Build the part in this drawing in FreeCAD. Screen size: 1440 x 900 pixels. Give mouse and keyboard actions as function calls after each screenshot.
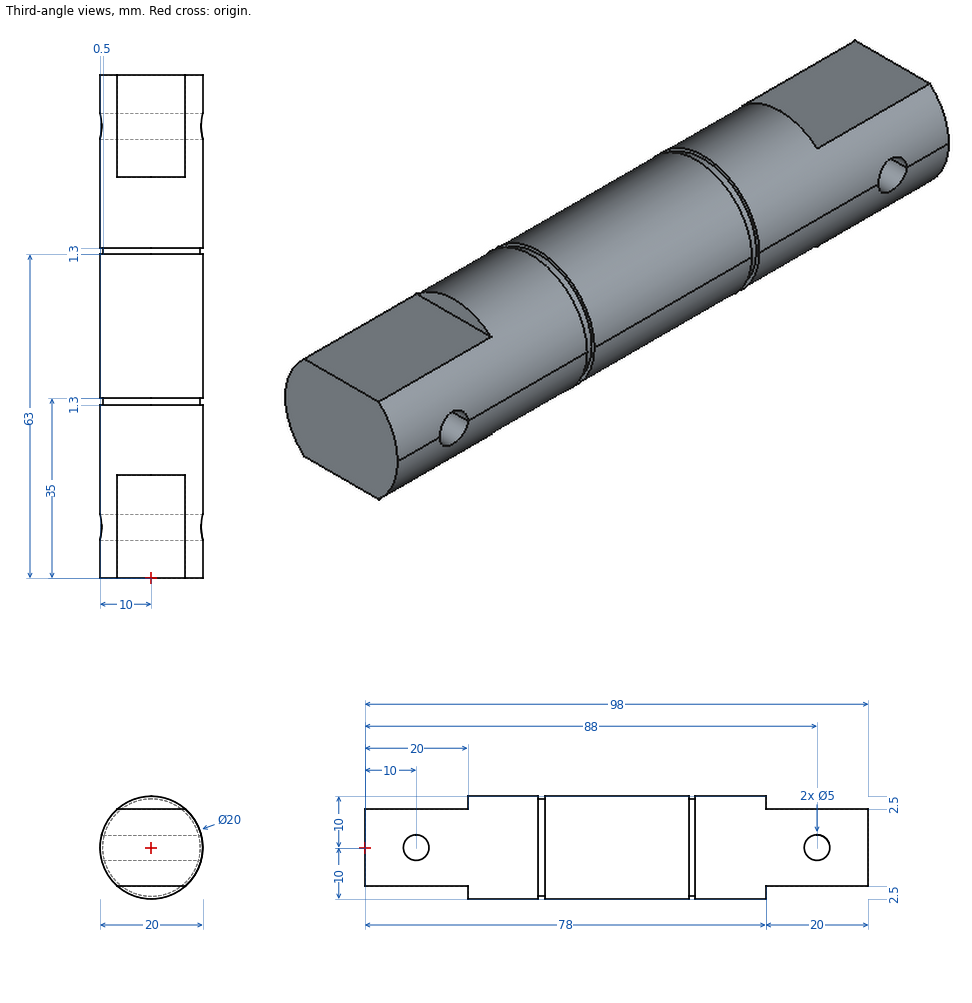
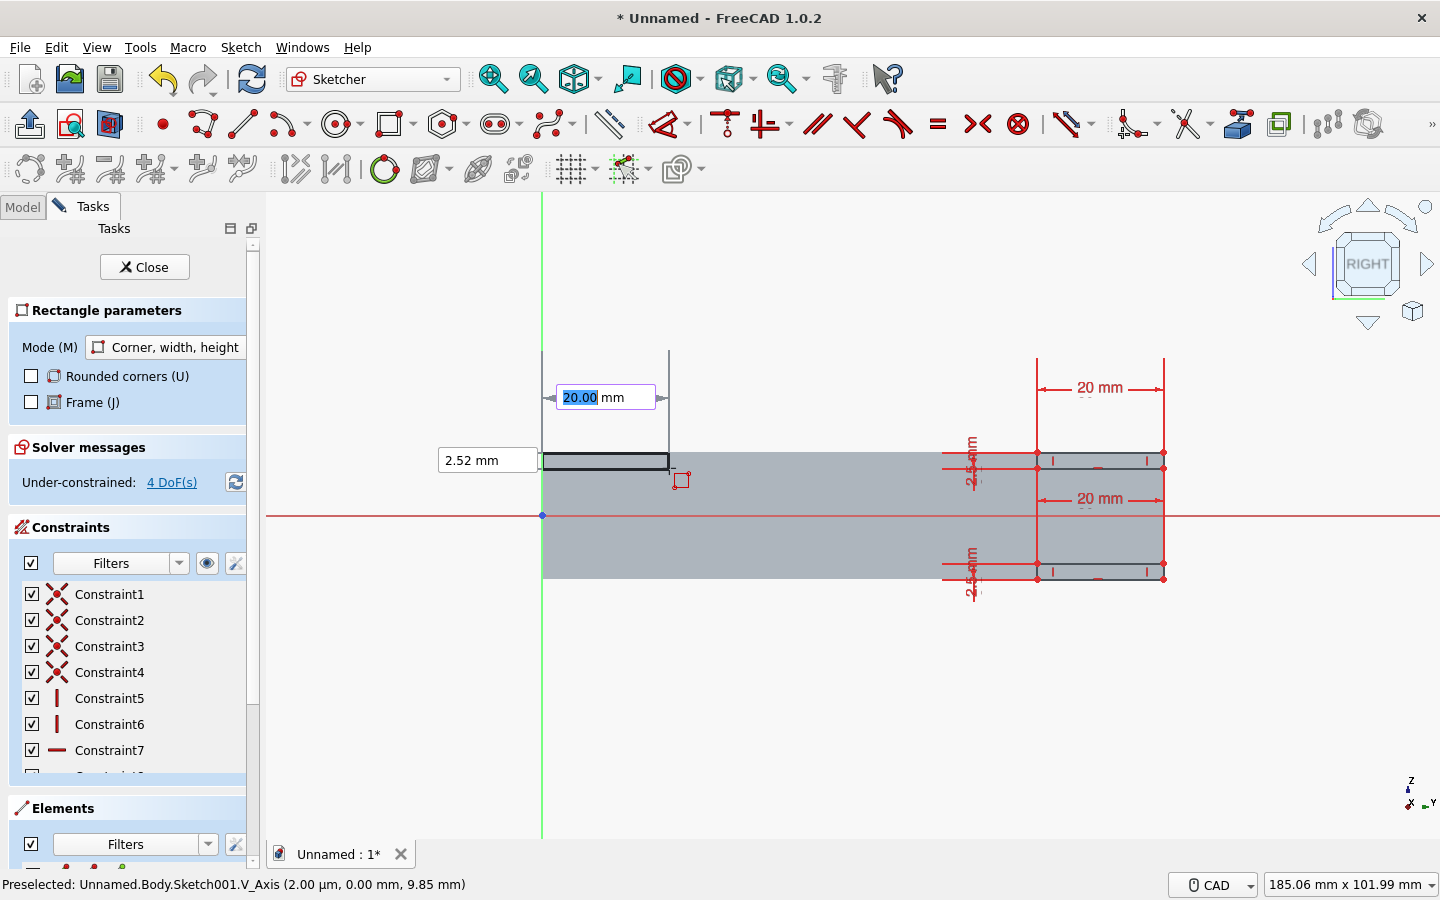
text(20)
key(Tab)
text(2.5)
key(Return)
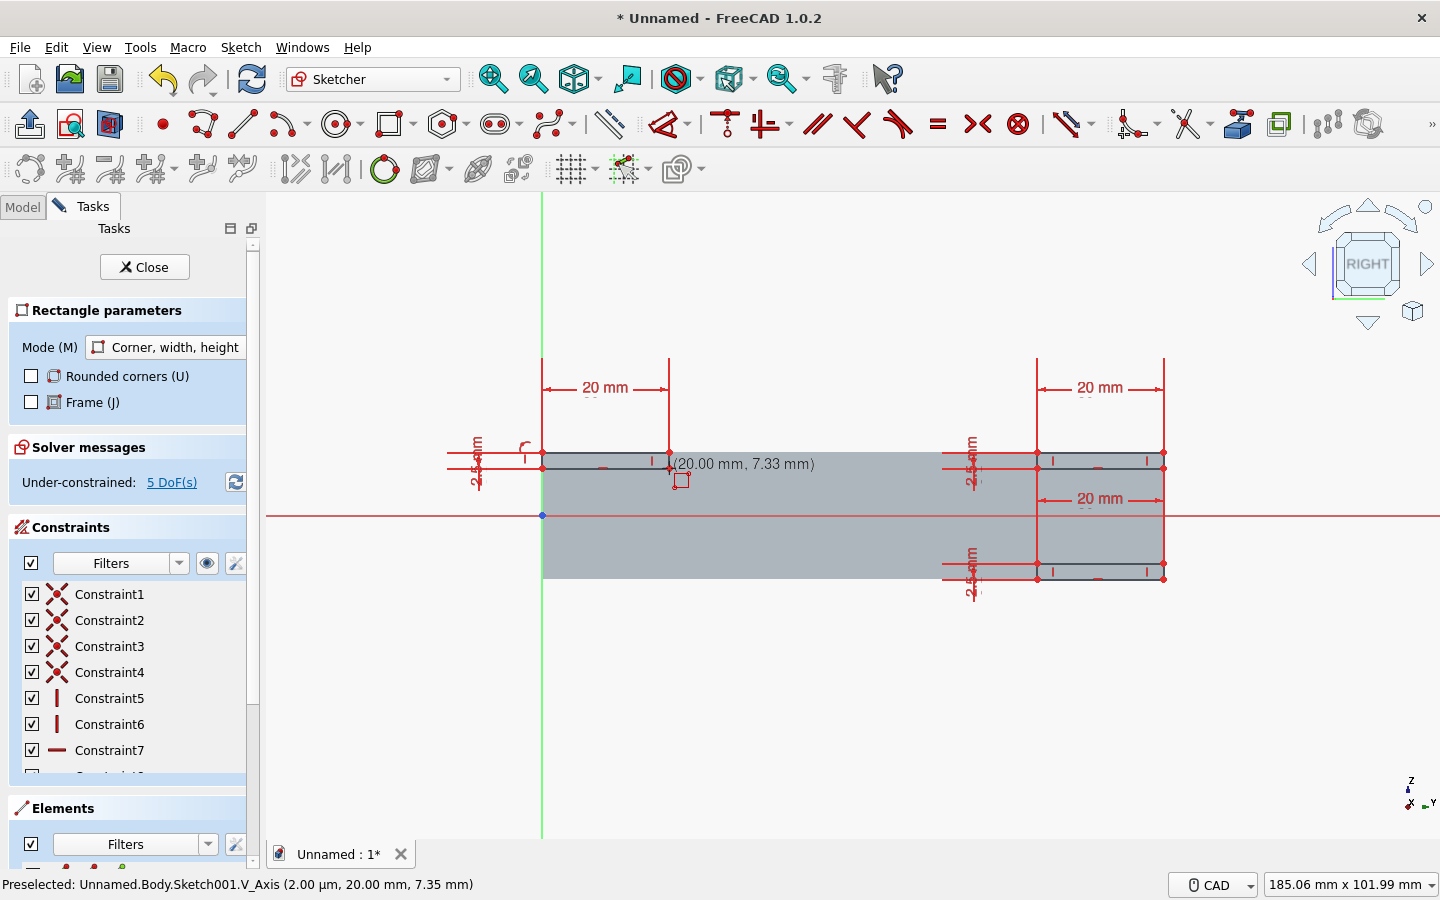
click(542, 563)
move(669, 579)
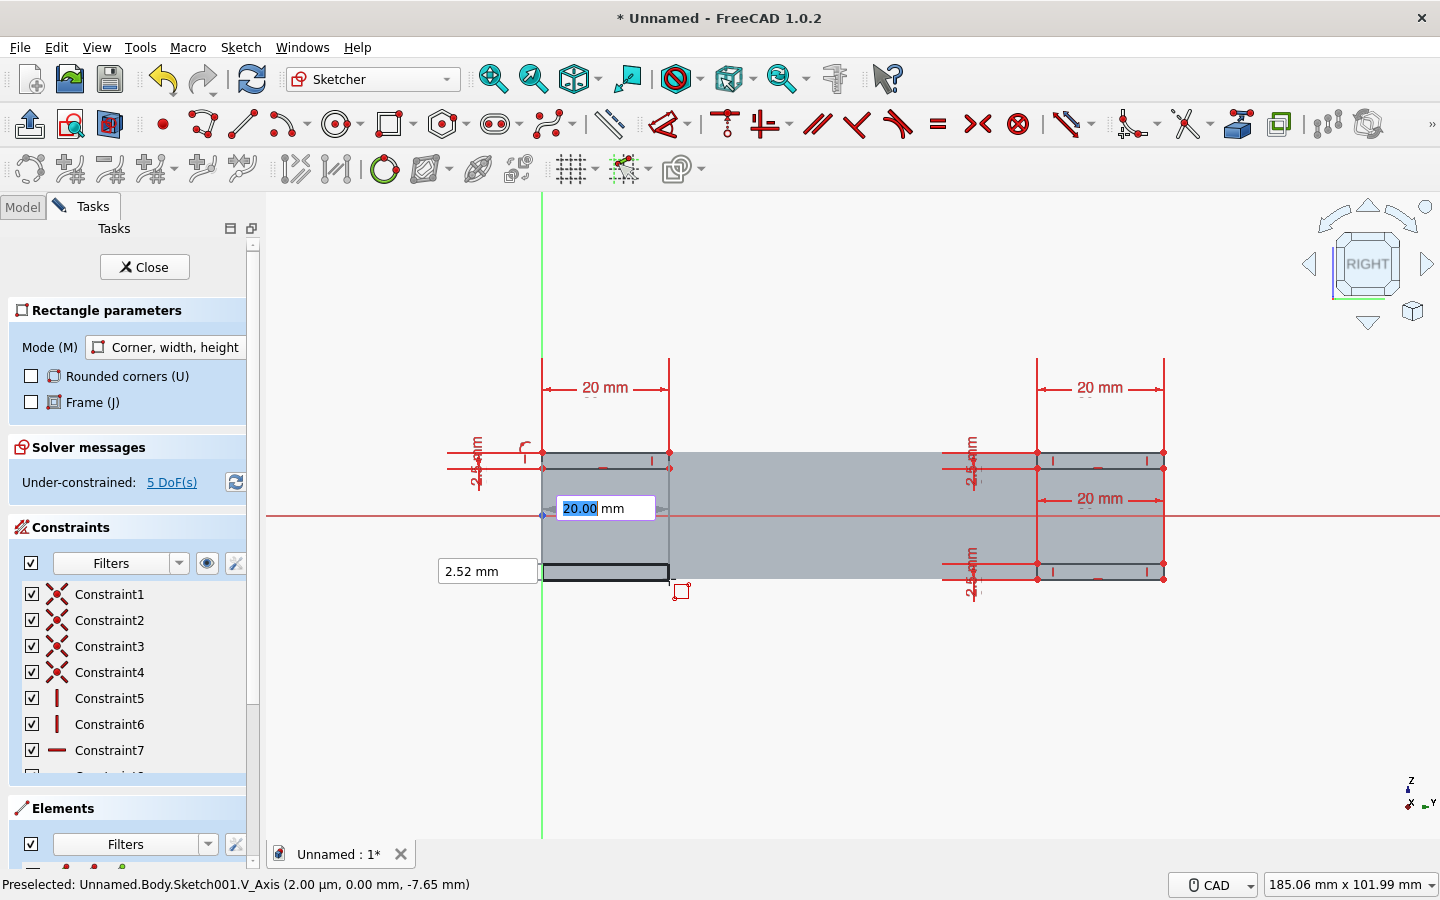
text(20)
key(Tab)
text(2.5)
key(Return)
key(Escape)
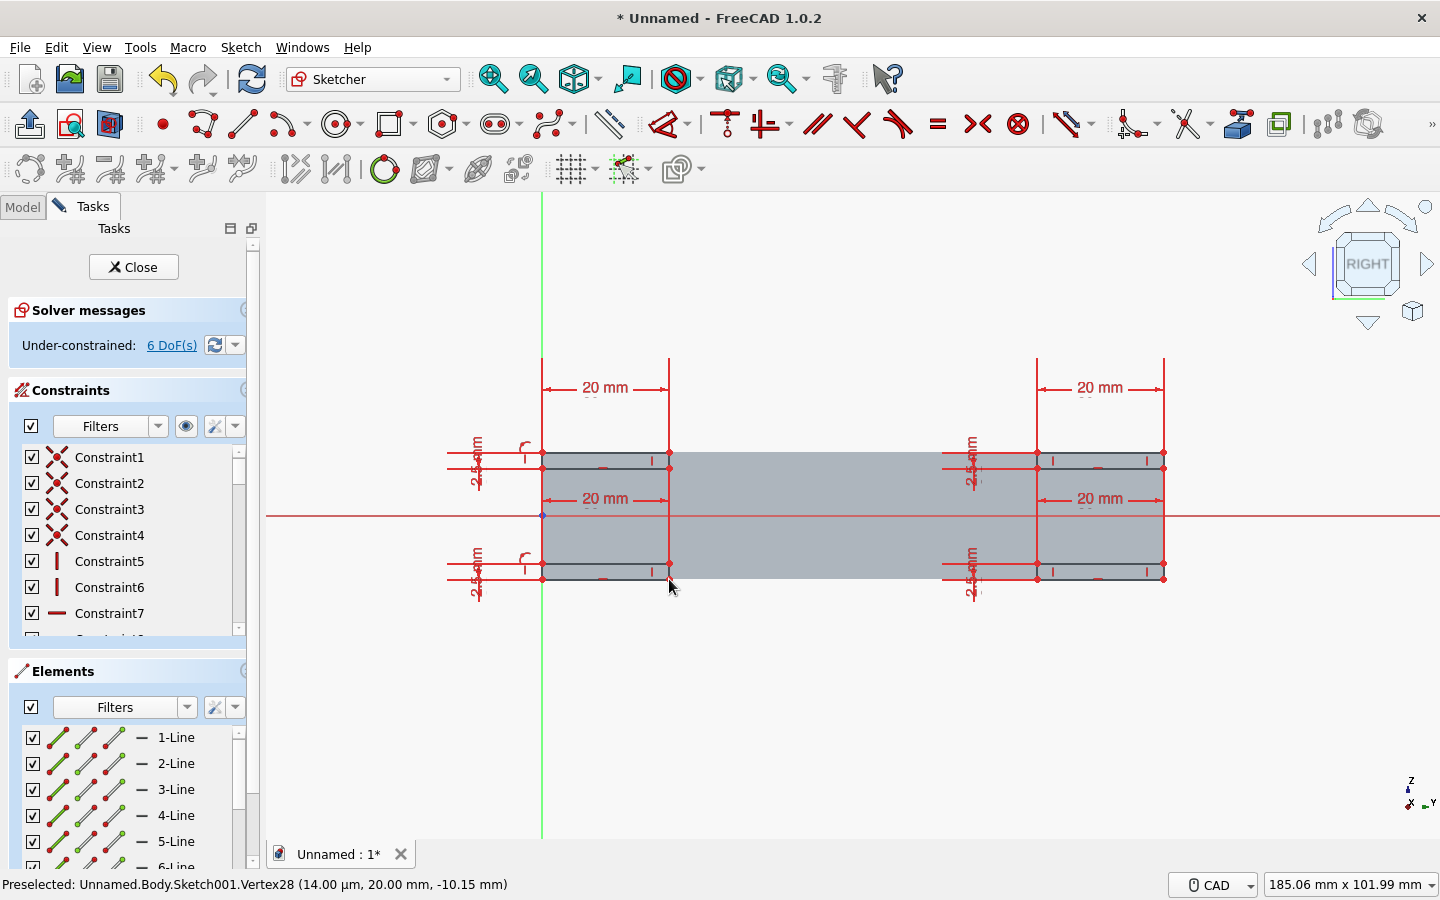
key(d)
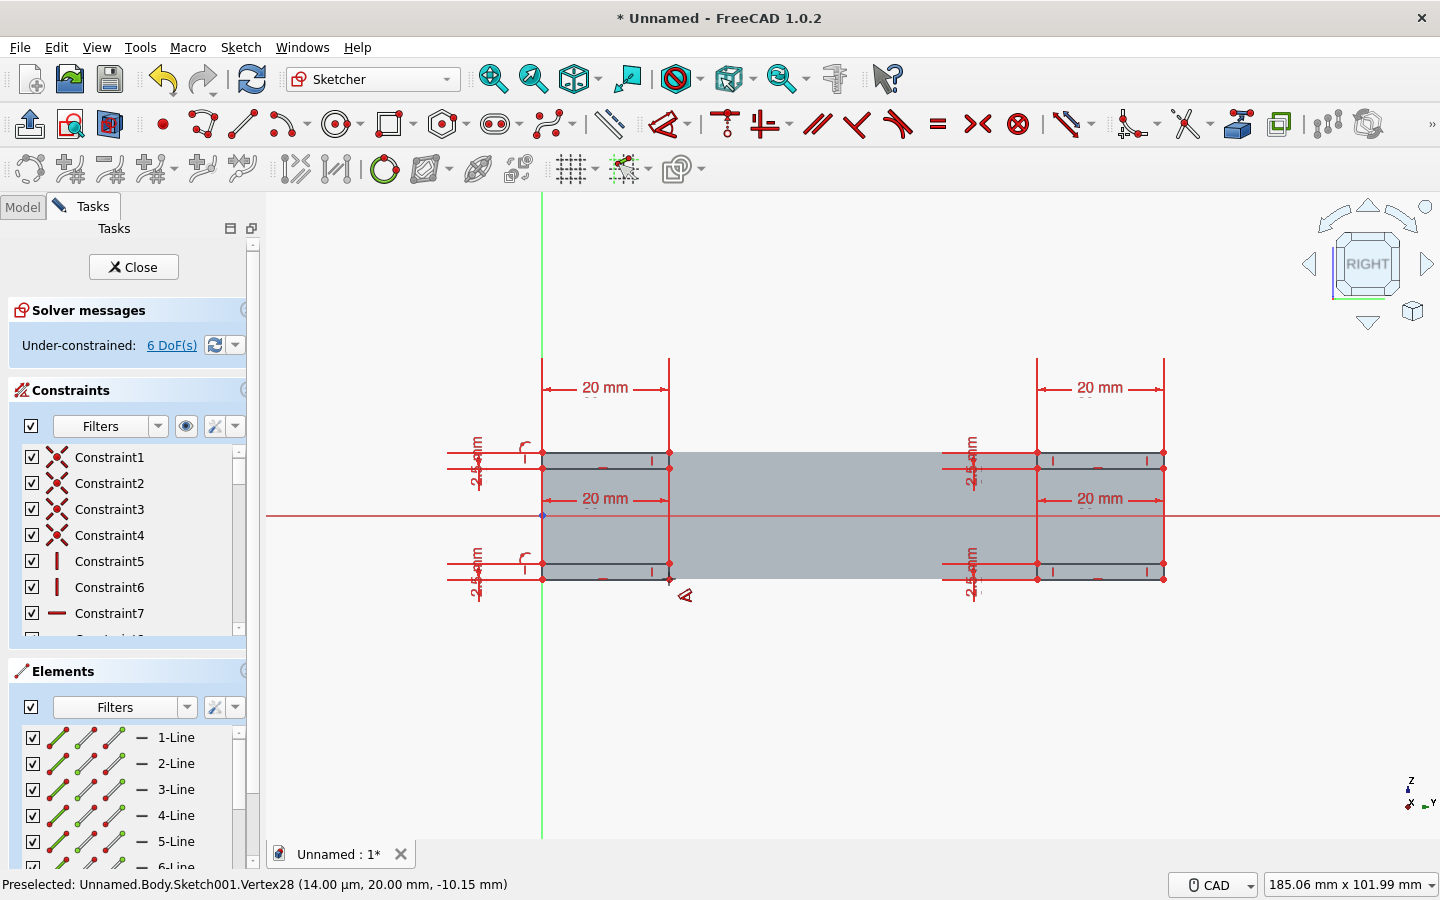
click(1037, 564)
click(790, 598)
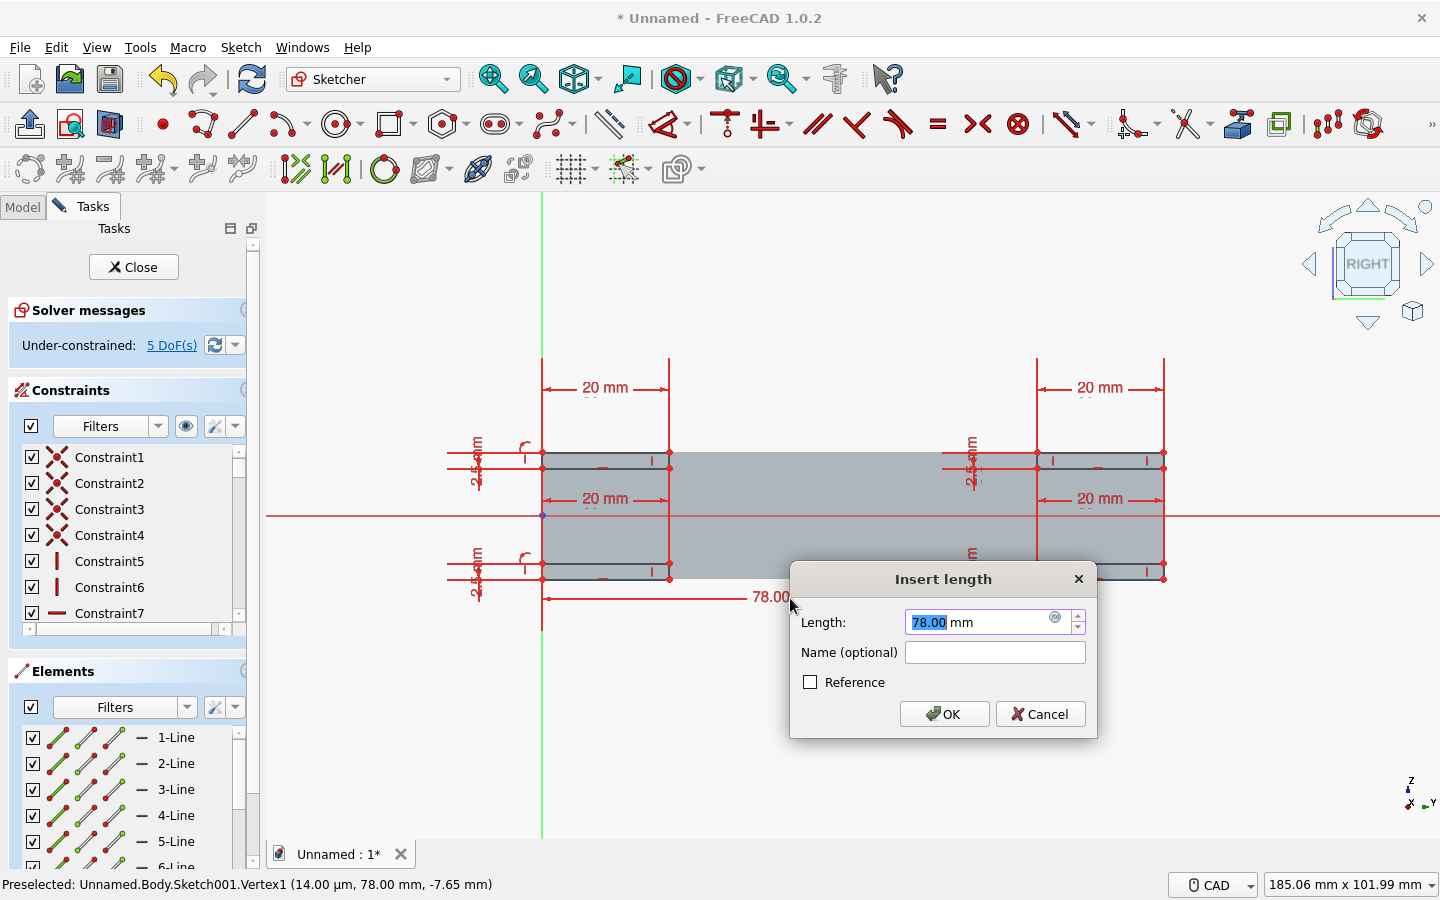
text(78)
key(Return)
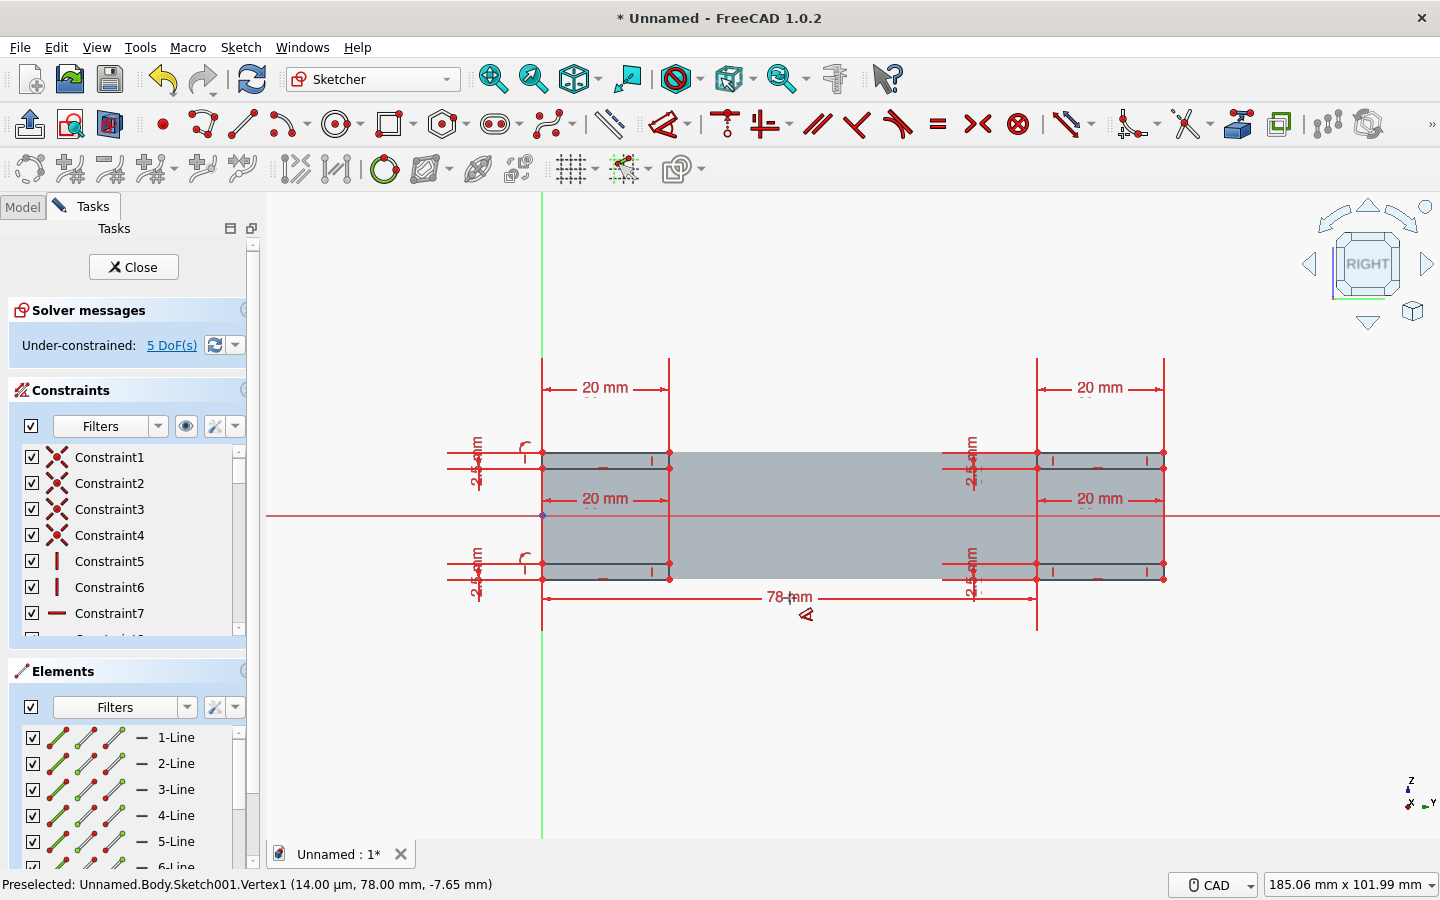
click(1037, 580)
click(508, 548)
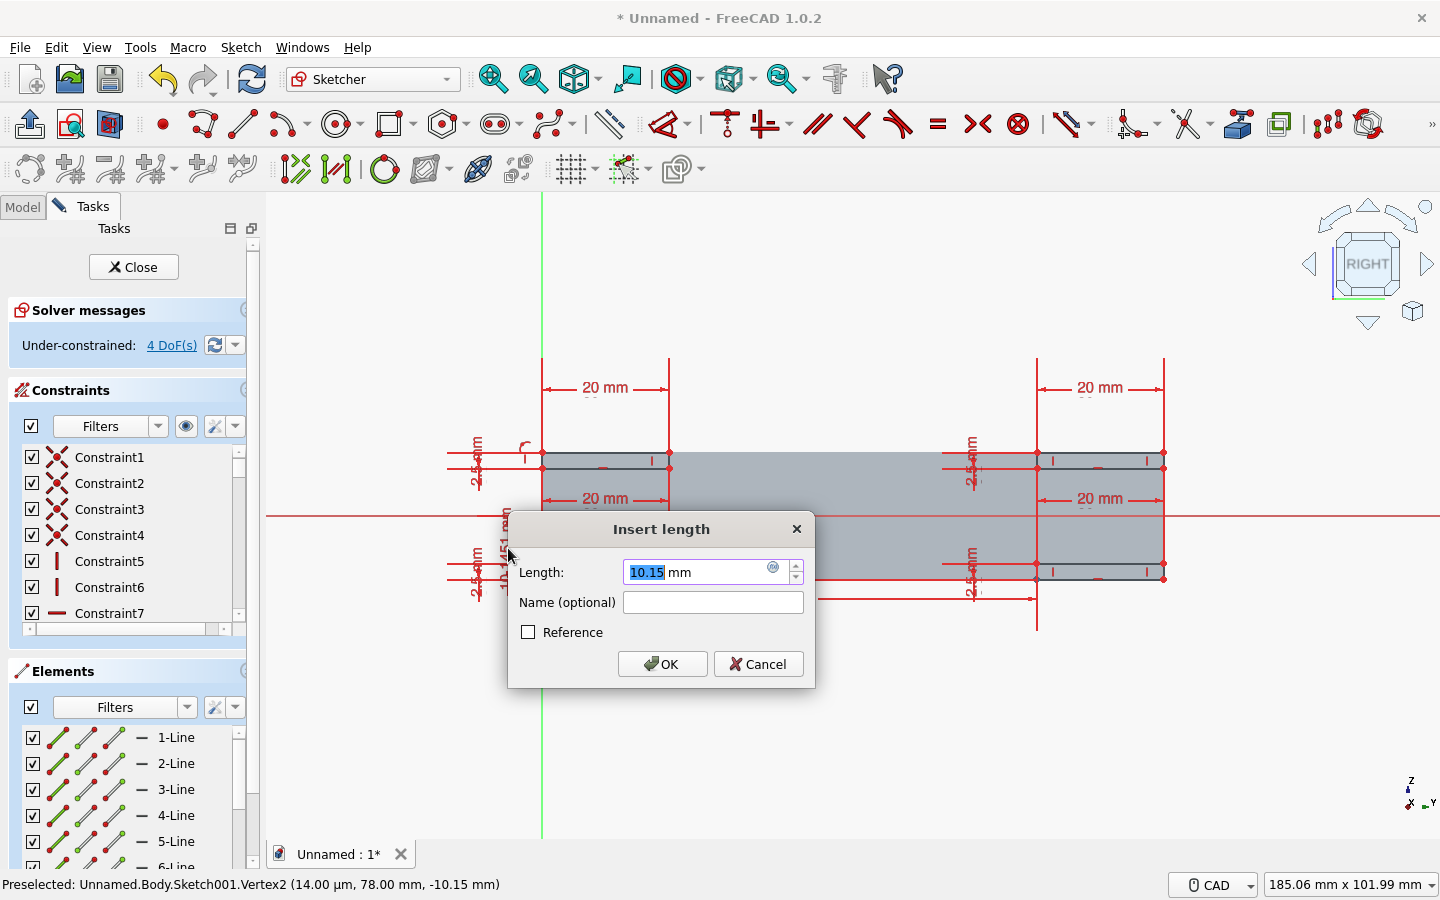
text(10)
key(Return)